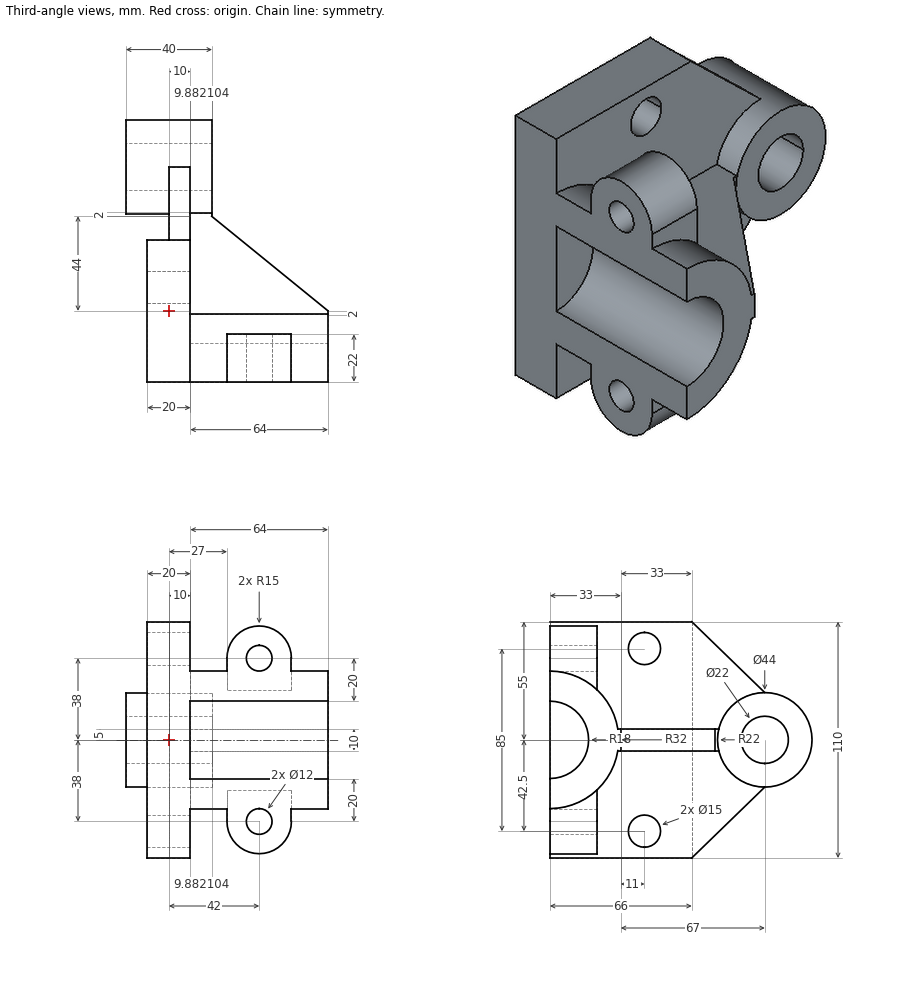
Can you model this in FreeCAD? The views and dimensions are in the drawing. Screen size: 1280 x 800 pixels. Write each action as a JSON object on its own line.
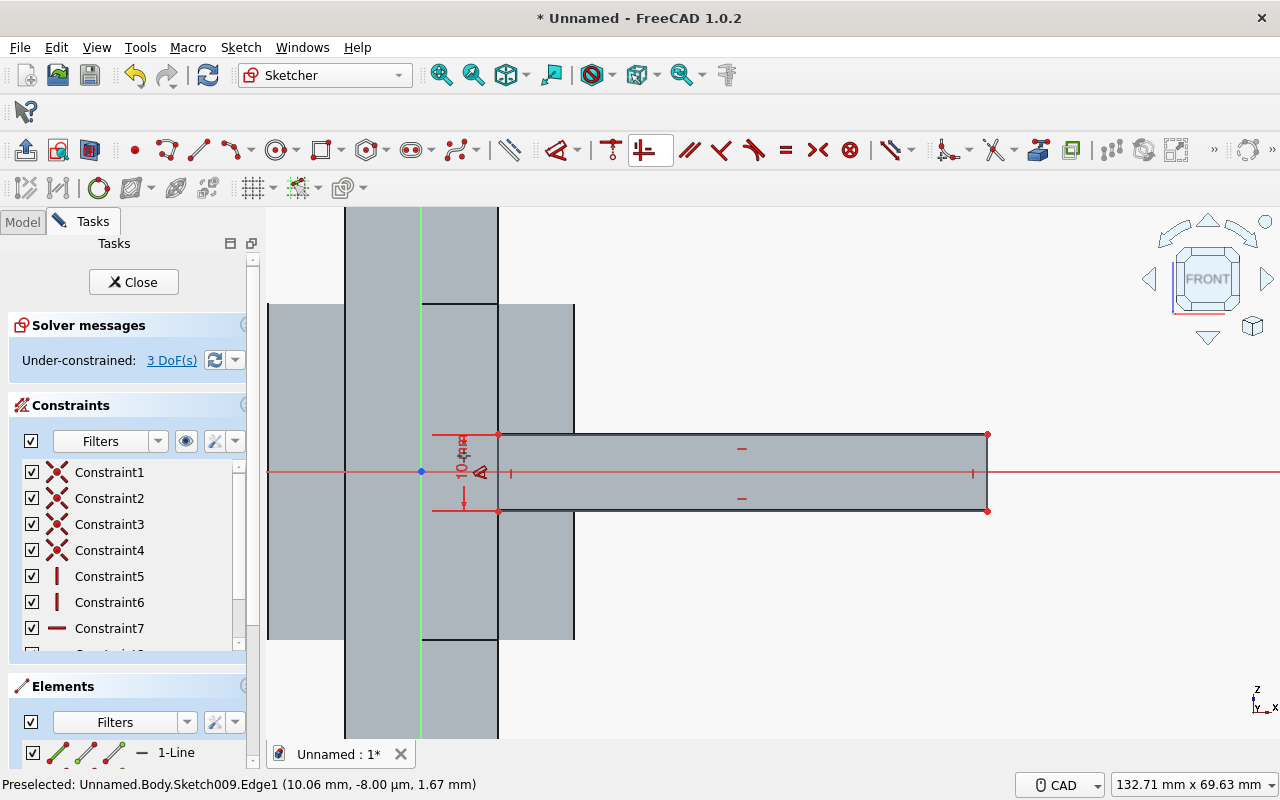
{"action": "left_click", "coordinate": [645, 511]}
{"action": "left_click", "coordinate": [743, 545]}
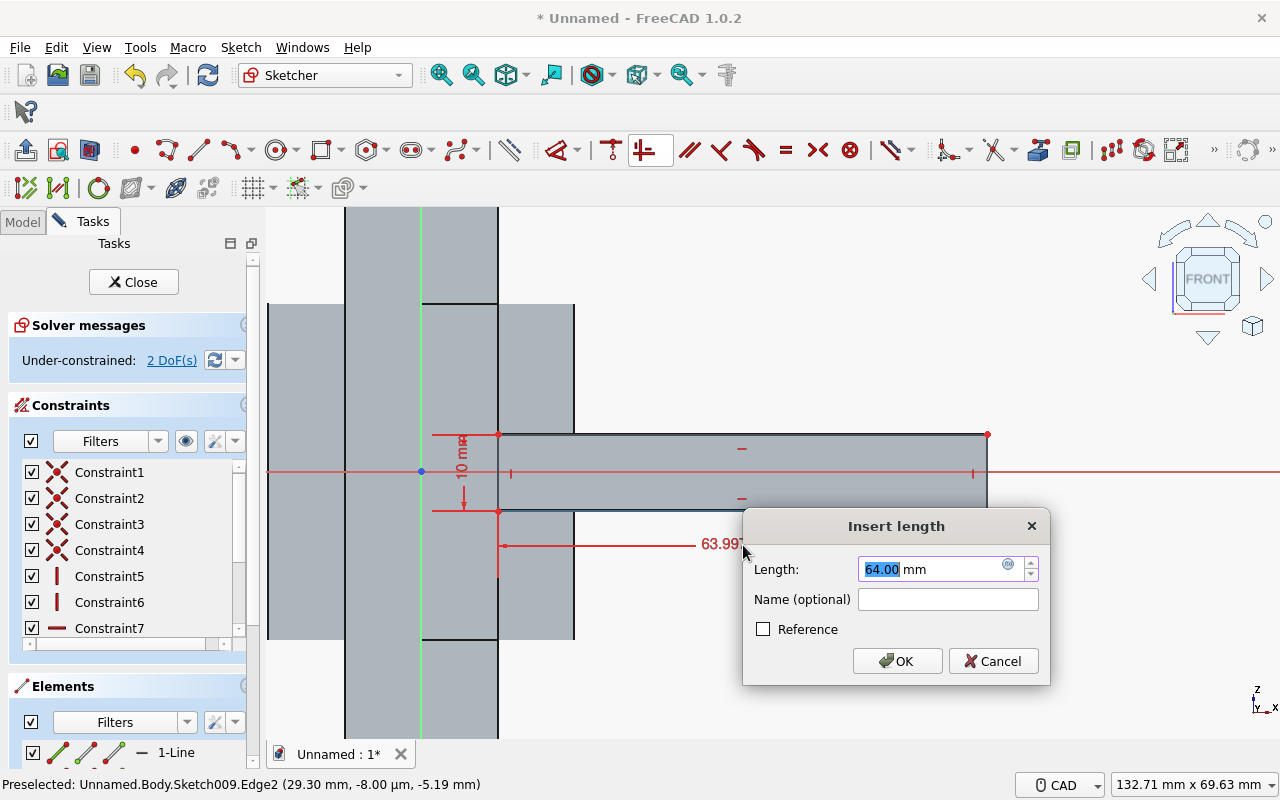
{"action": "type", "text": "64"}
{"action": "key", "text": "Return"}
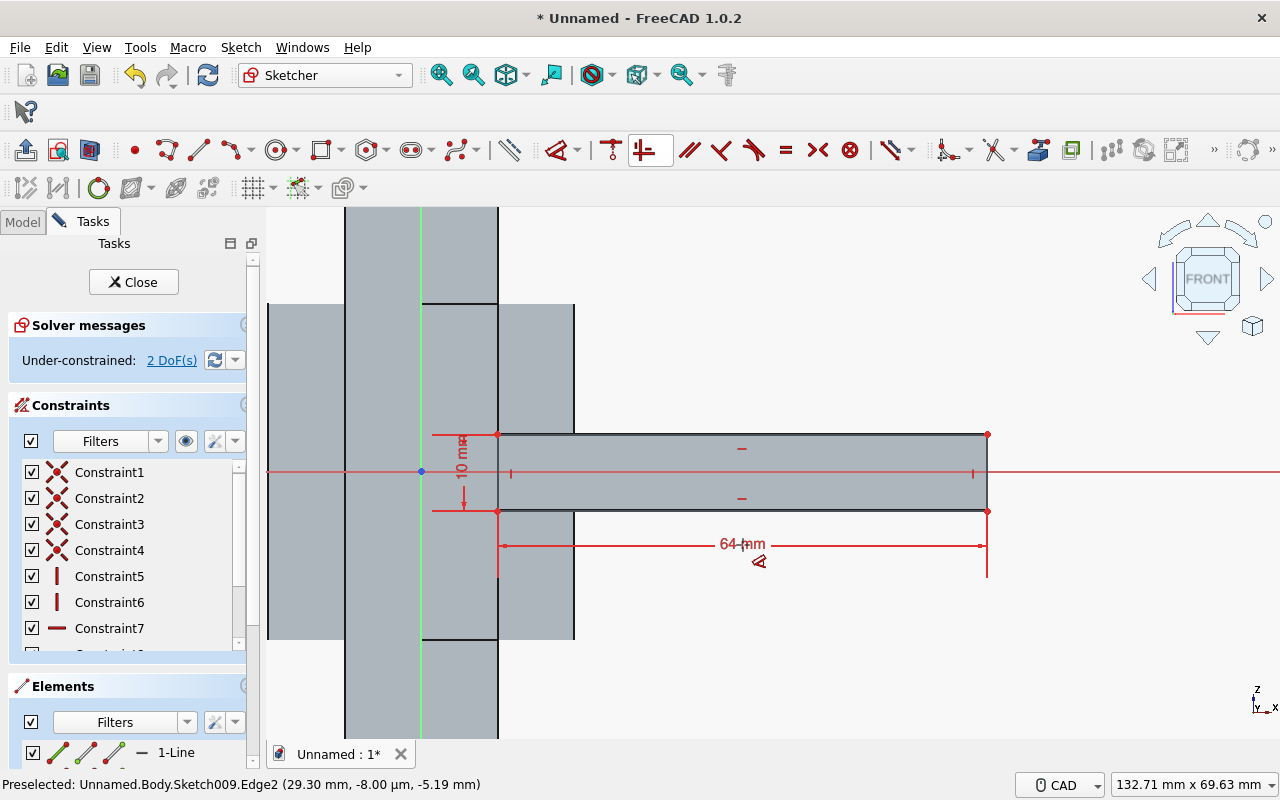
{"action": "left_click", "coordinate": [498, 435]}
{"action": "left_click", "coordinate": [387, 453]}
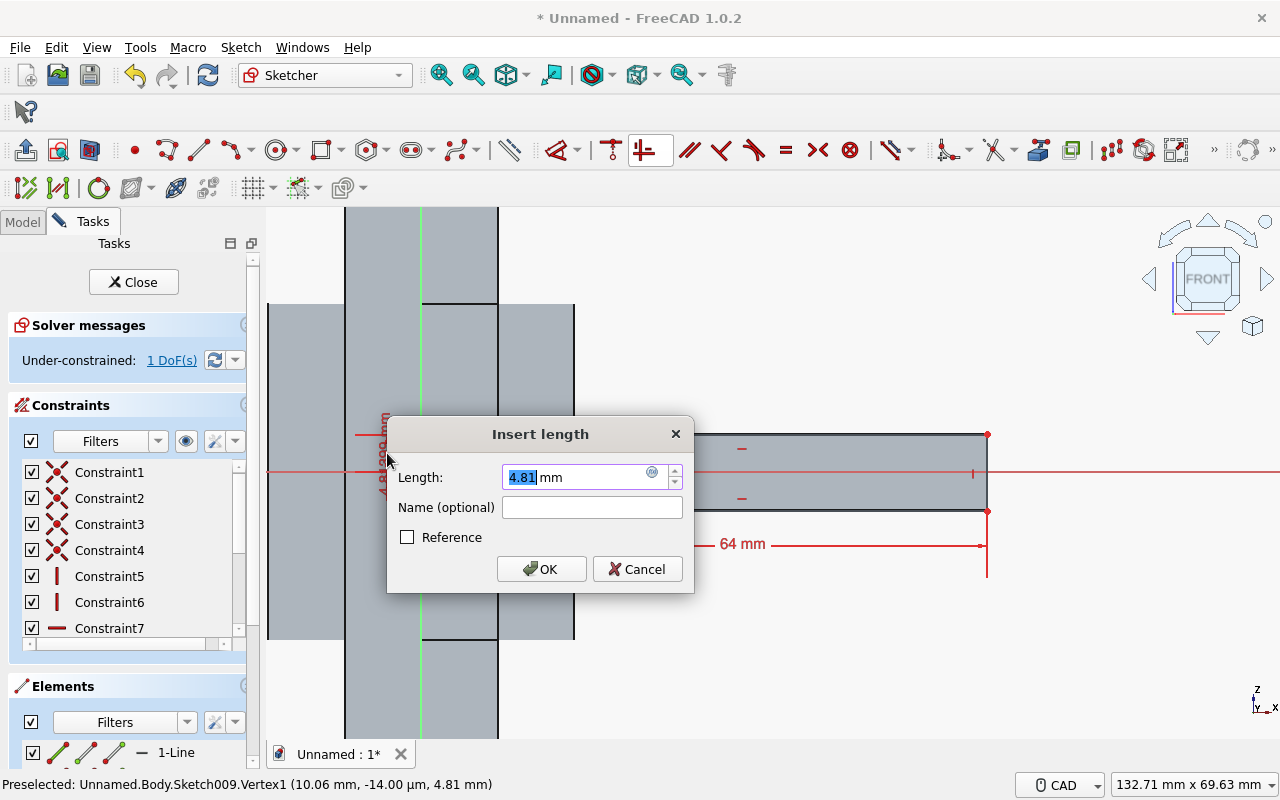
{"action": "type", "text": "5"}
{"action": "key", "text": "Return"}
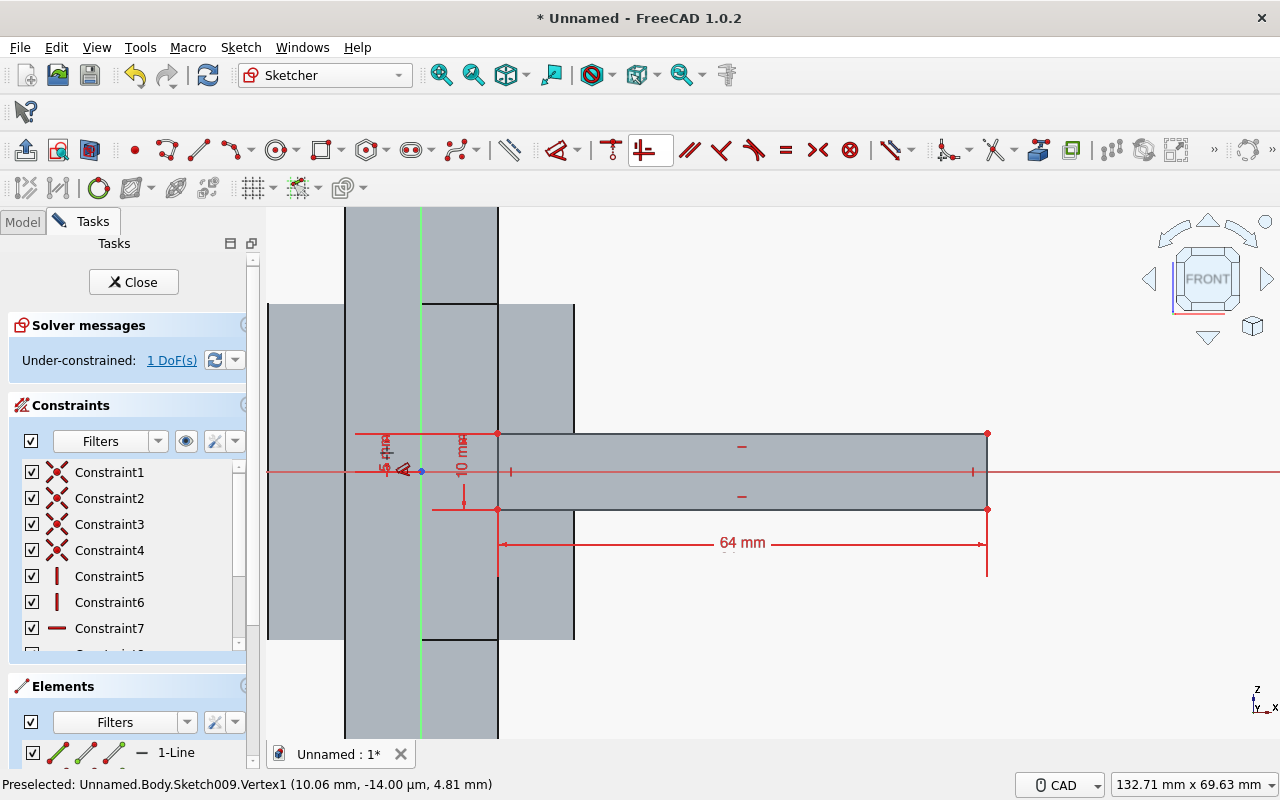
{"action": "left_click", "coordinate": [498, 434]}
{"action": "left_click", "coordinate": [460, 400]}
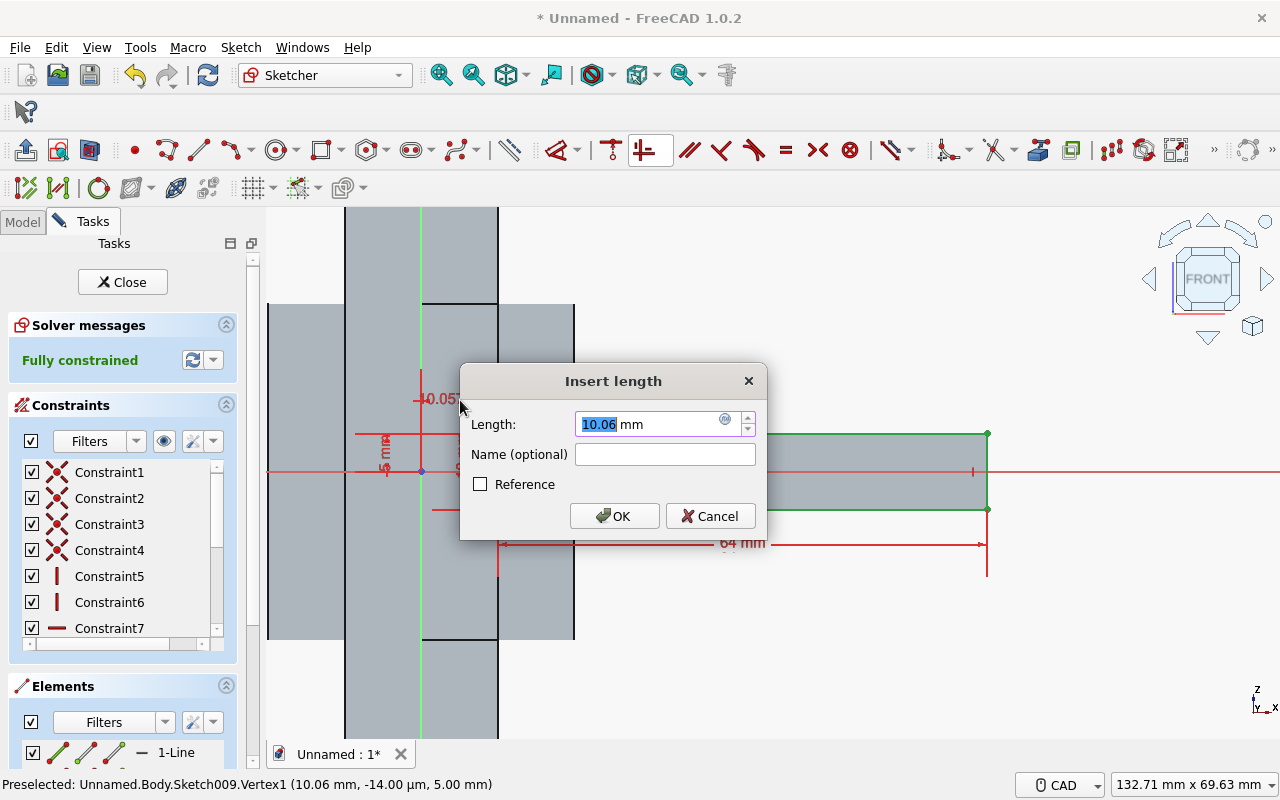
{"action": "type", "text": "10"}
{"action": "key", "text": "Return"}
{"action": "key", "text": "Escape"}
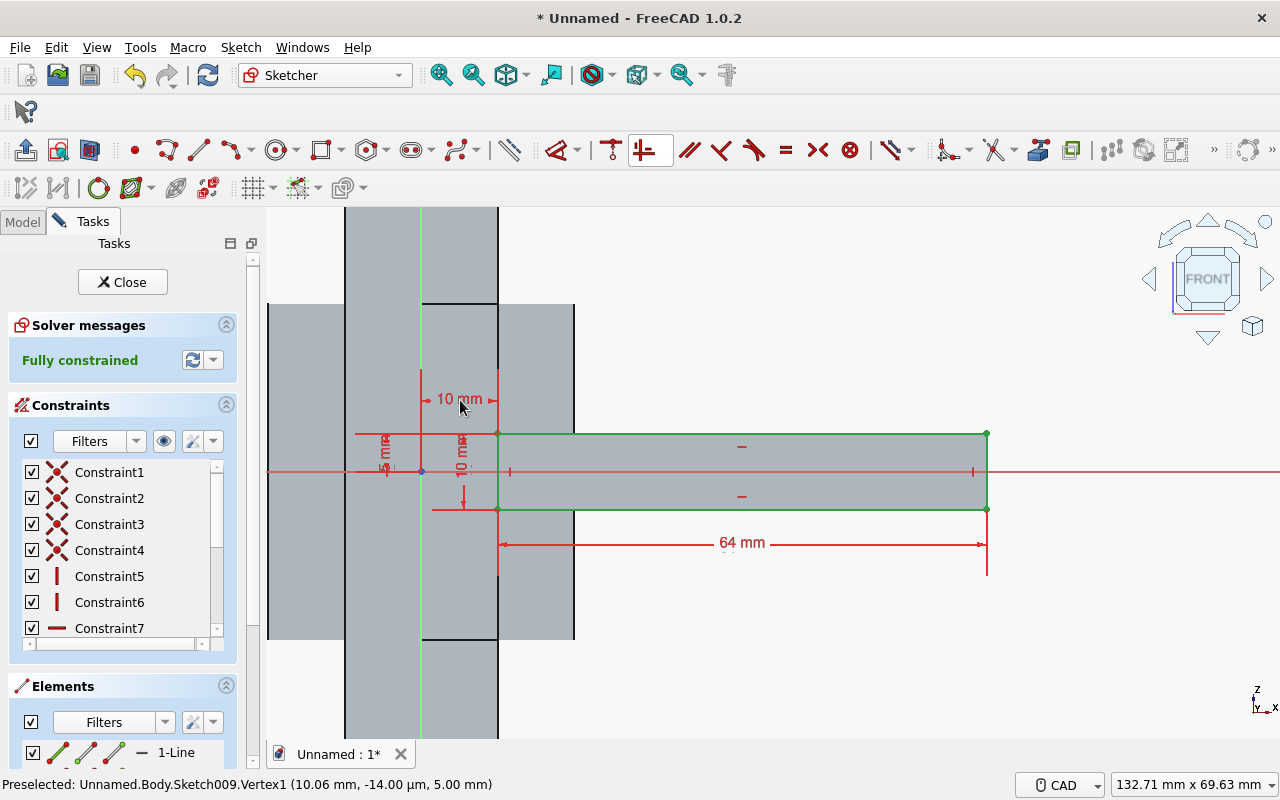
{"action": "left_click", "coordinate": [123, 282]}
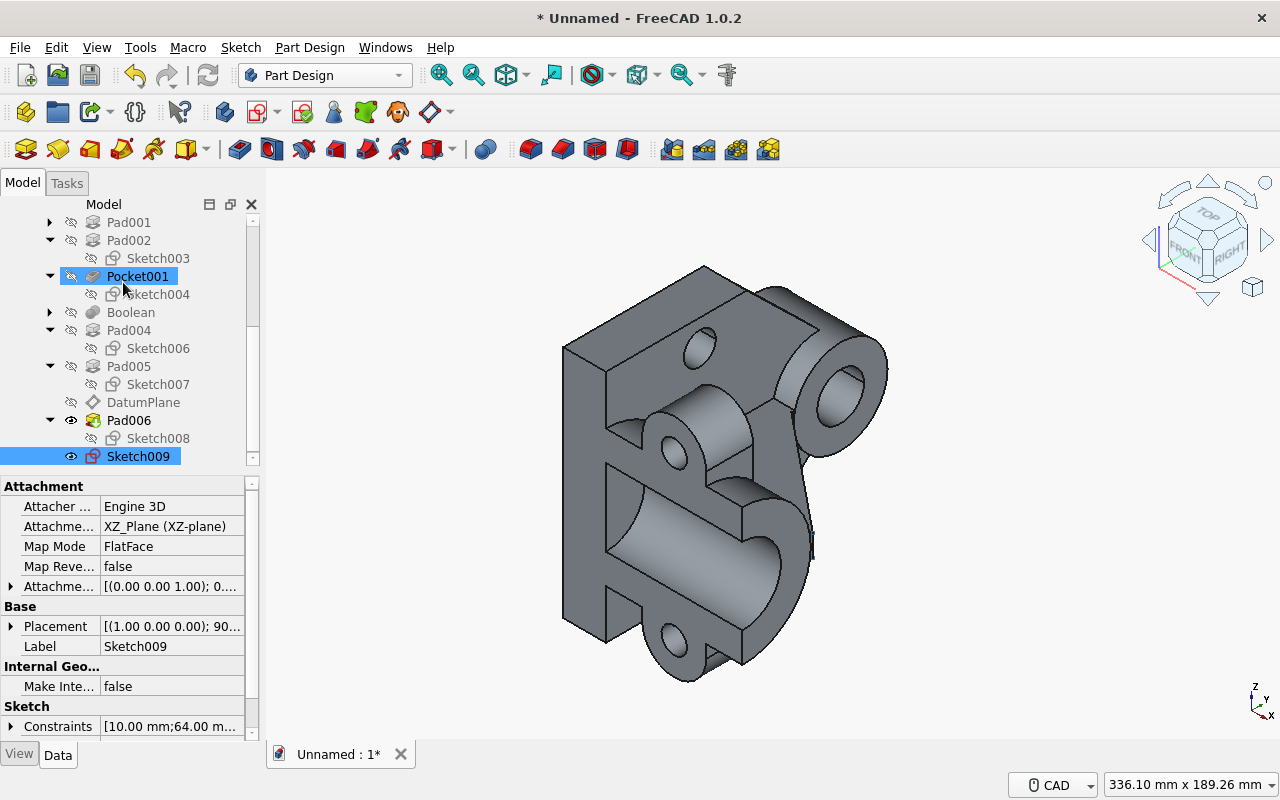
{"action": "left_click", "coordinate": [26, 150]}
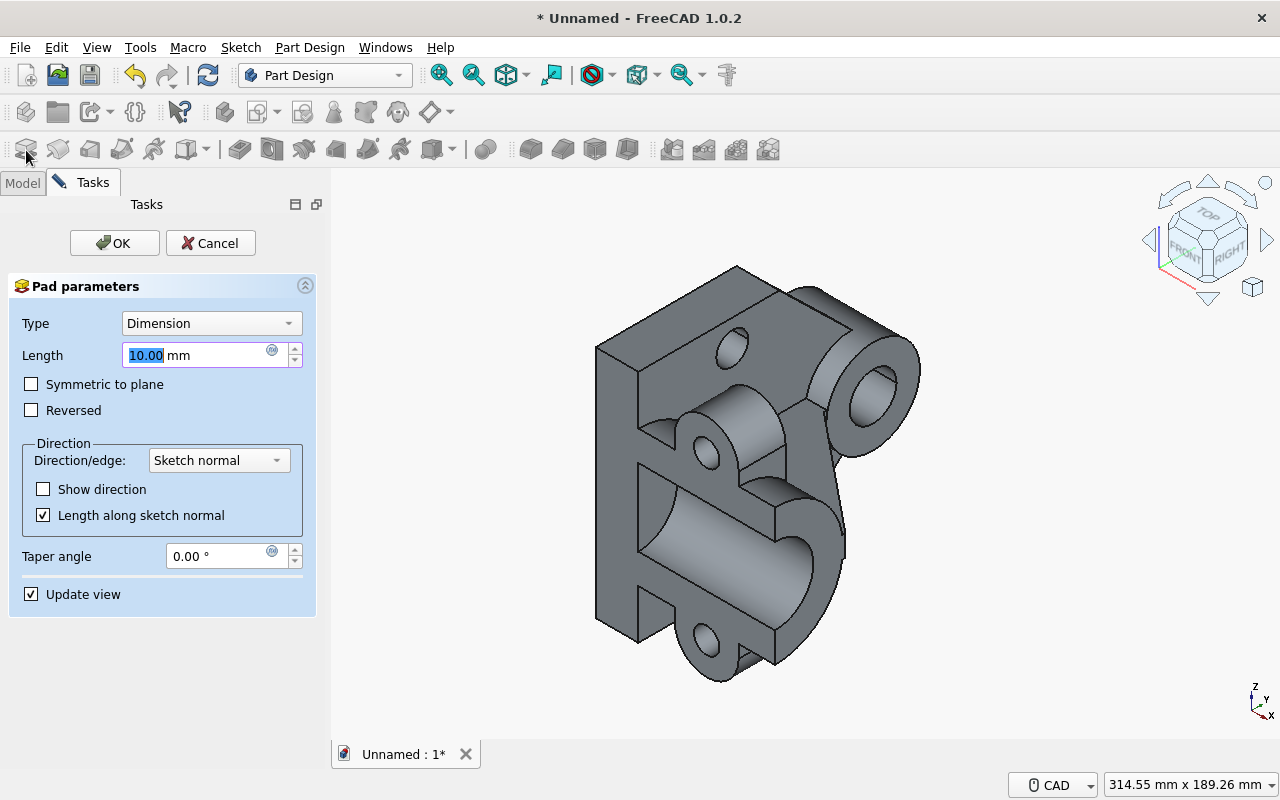
{"action": "type", "text": "2"}
{"action": "key", "text": "Tab"}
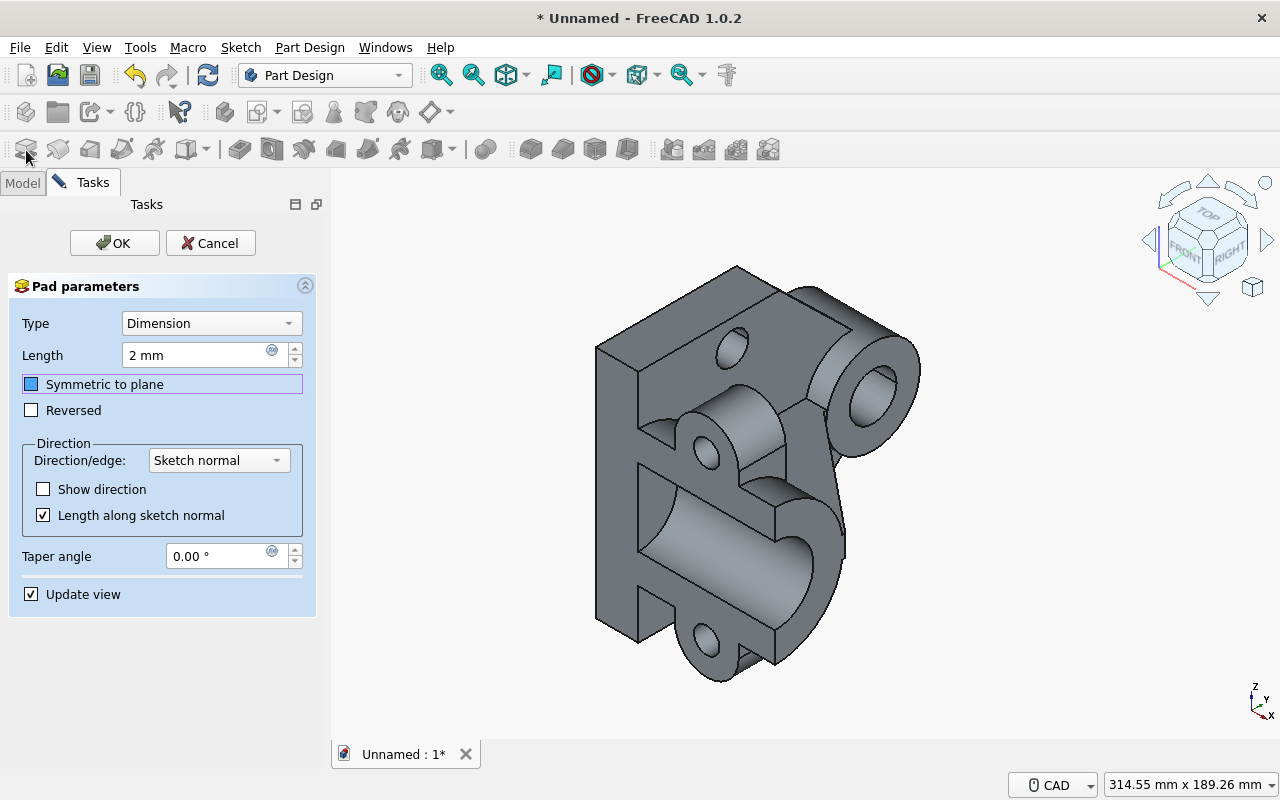
{"action": "left_click", "coordinate": [115, 243]}